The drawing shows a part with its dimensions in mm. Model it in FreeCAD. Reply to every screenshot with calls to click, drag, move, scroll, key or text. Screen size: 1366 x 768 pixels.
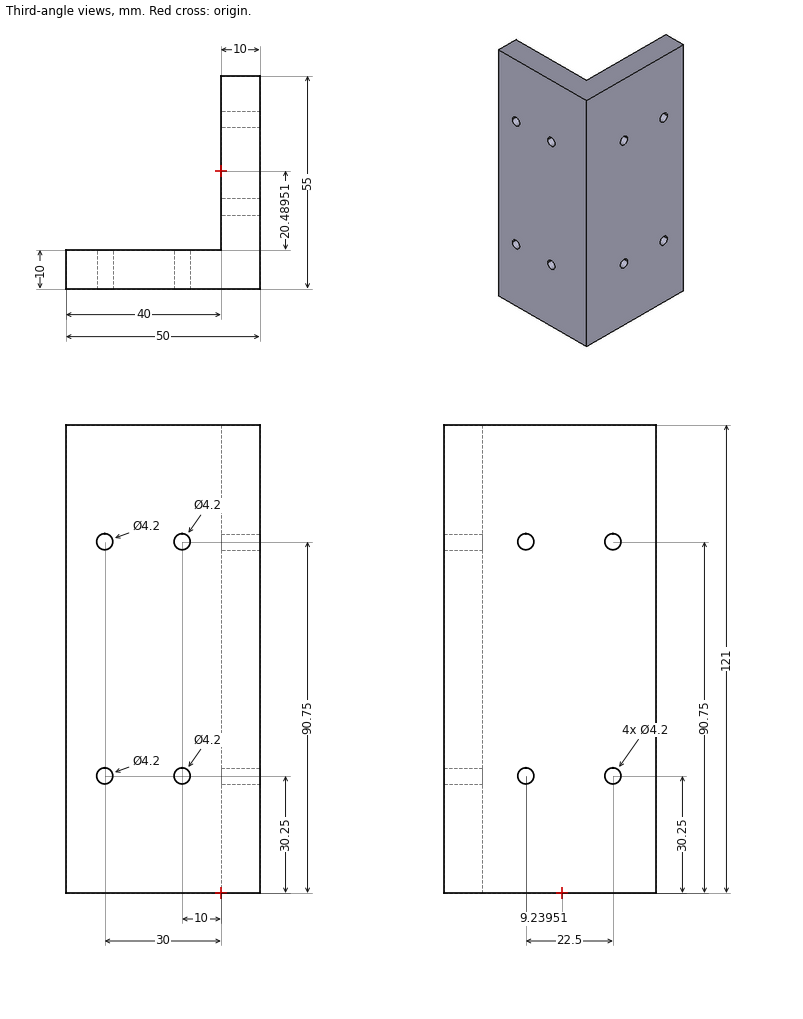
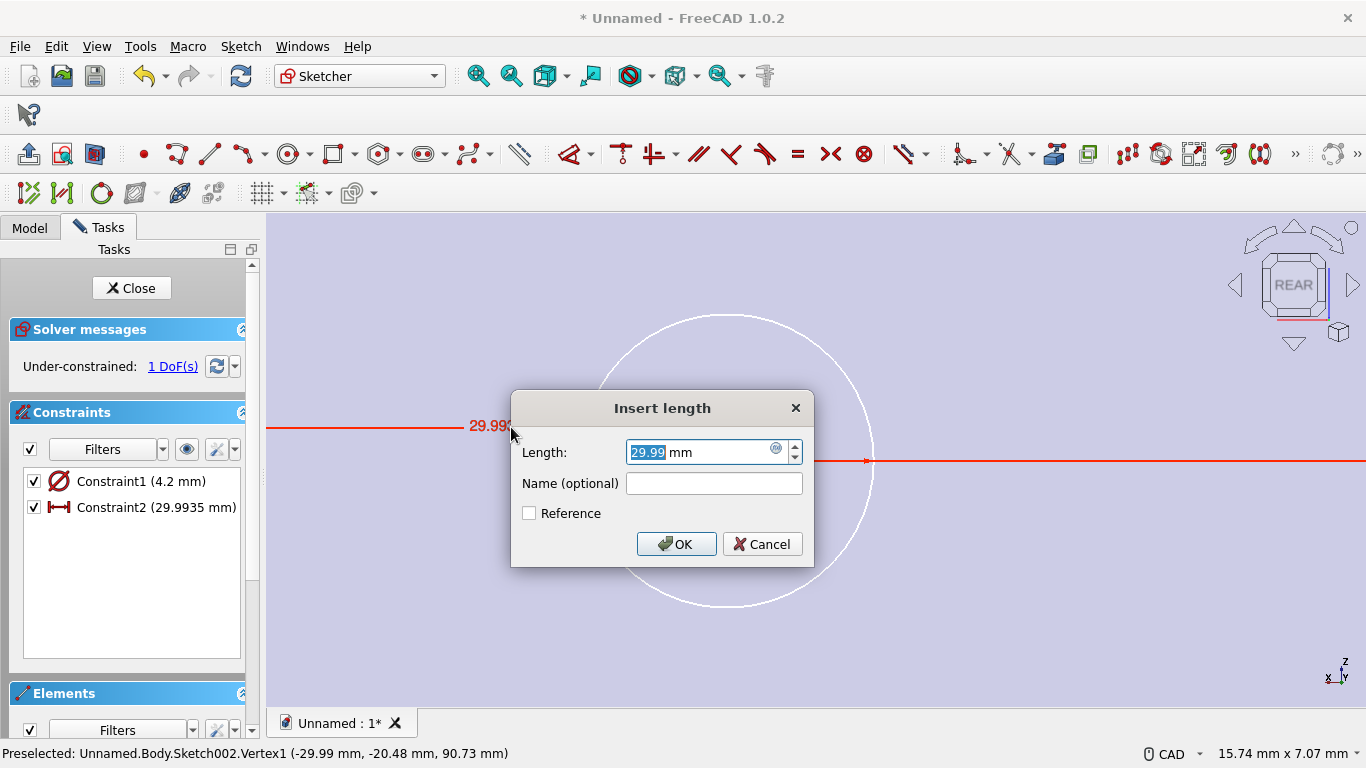
text(30)
key(Return)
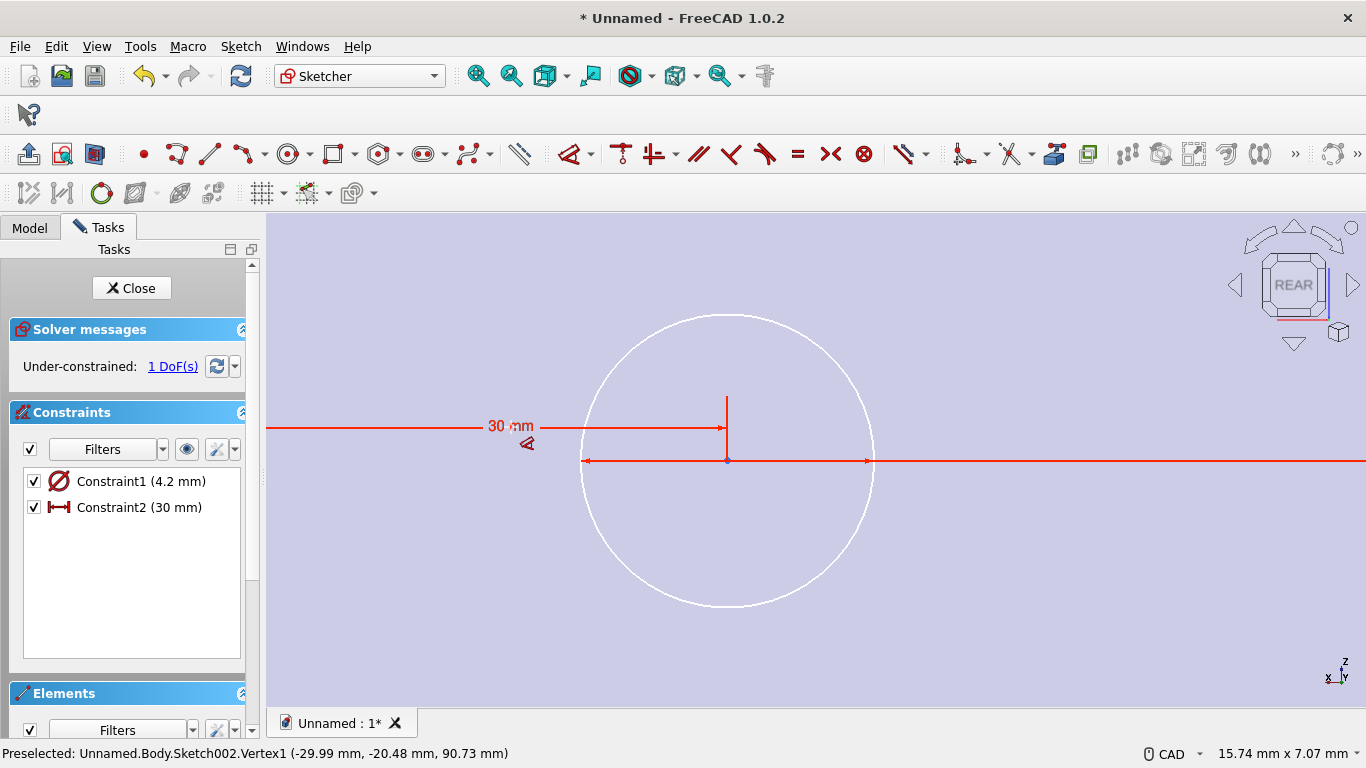
click(727, 461)
click(761, 570)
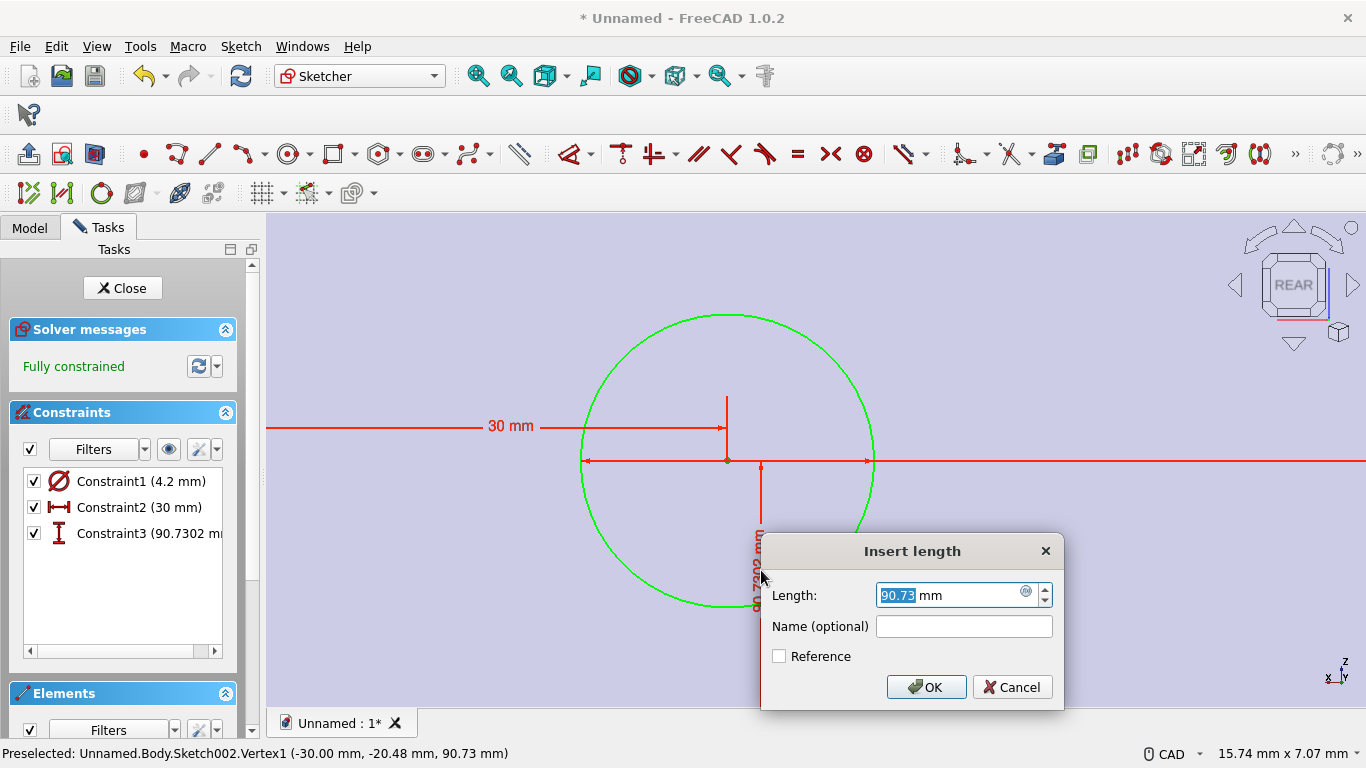
text(90.75)
key(Return)
key(Escape)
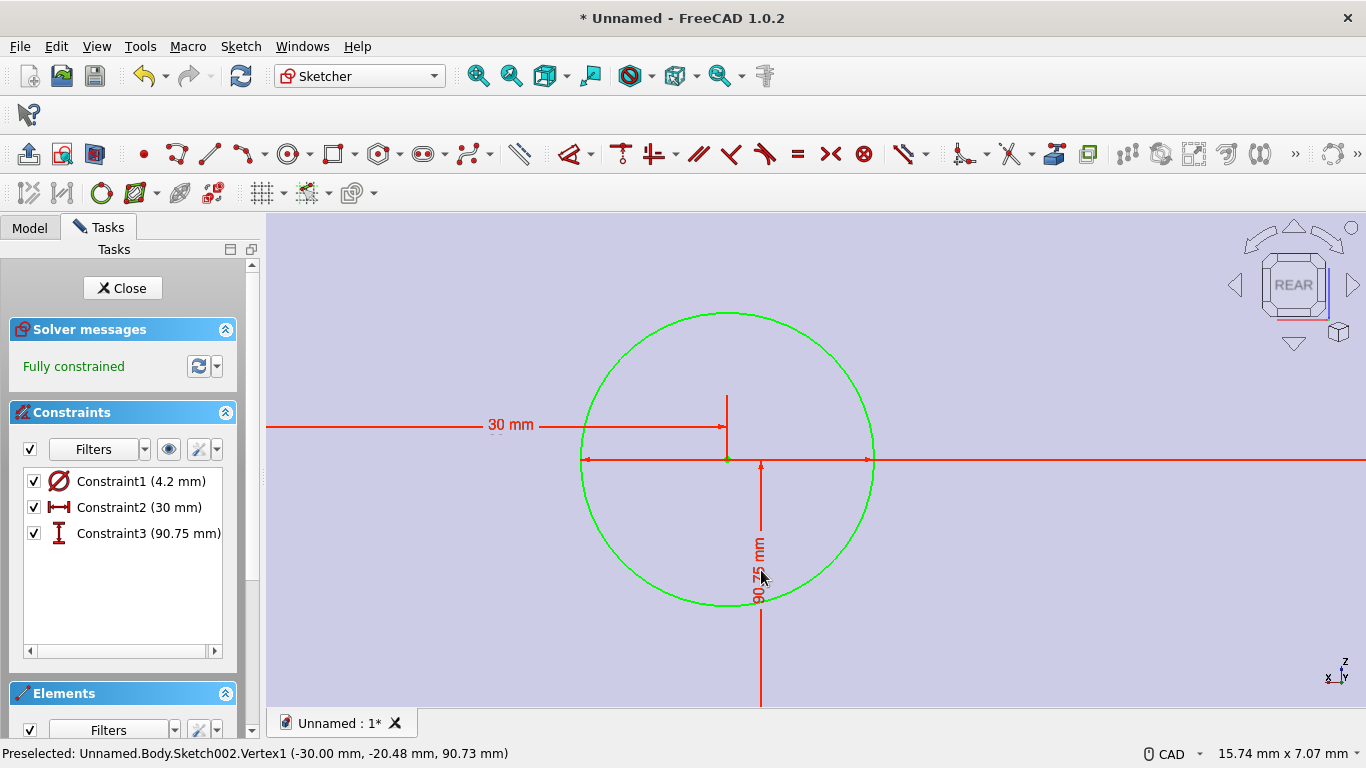
click(123, 288)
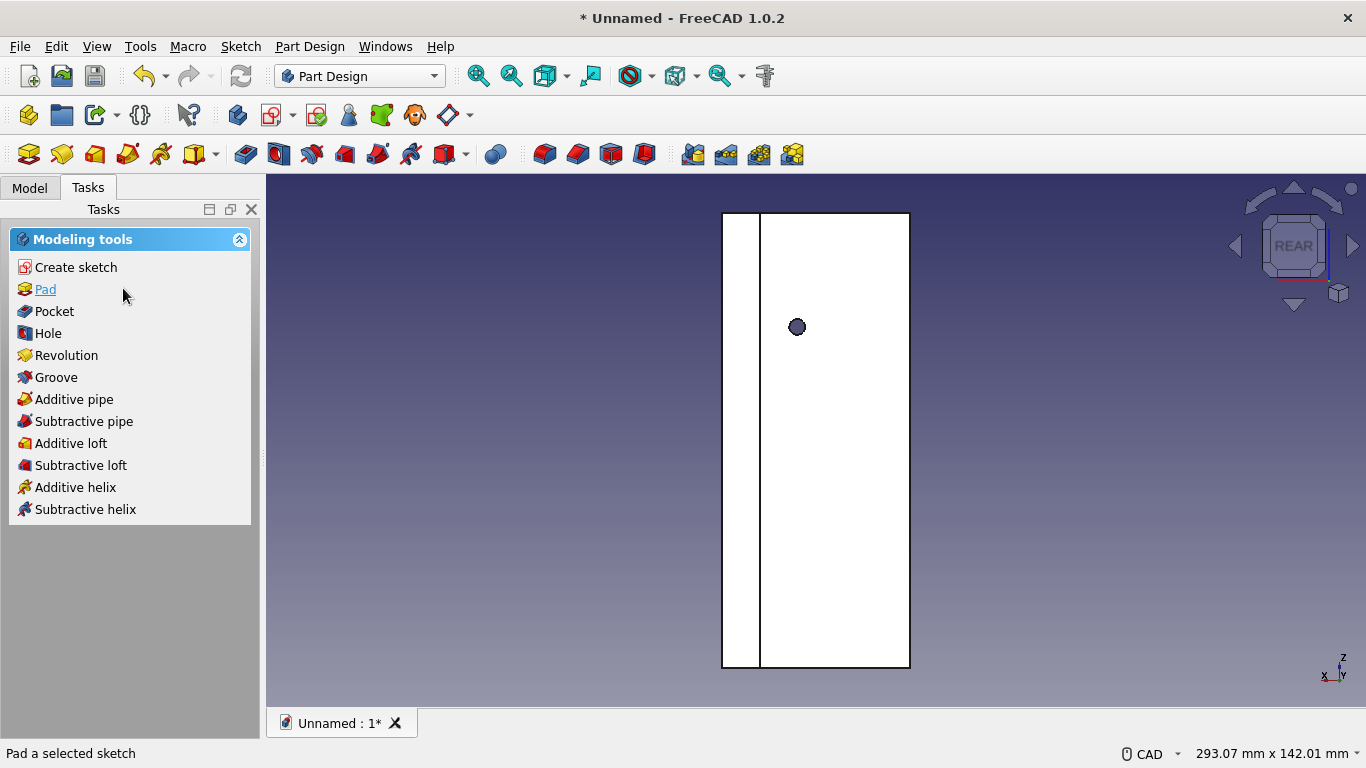
click(246, 154)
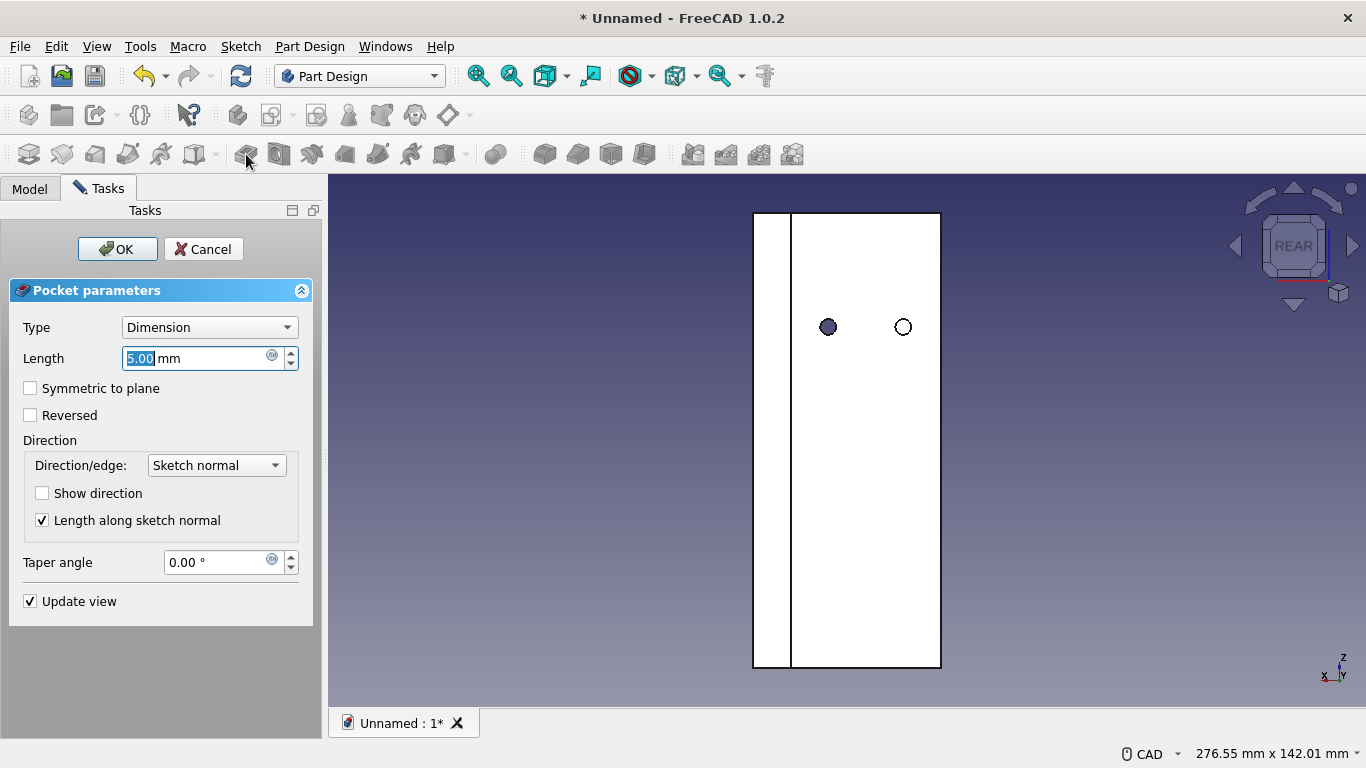
click(210, 328)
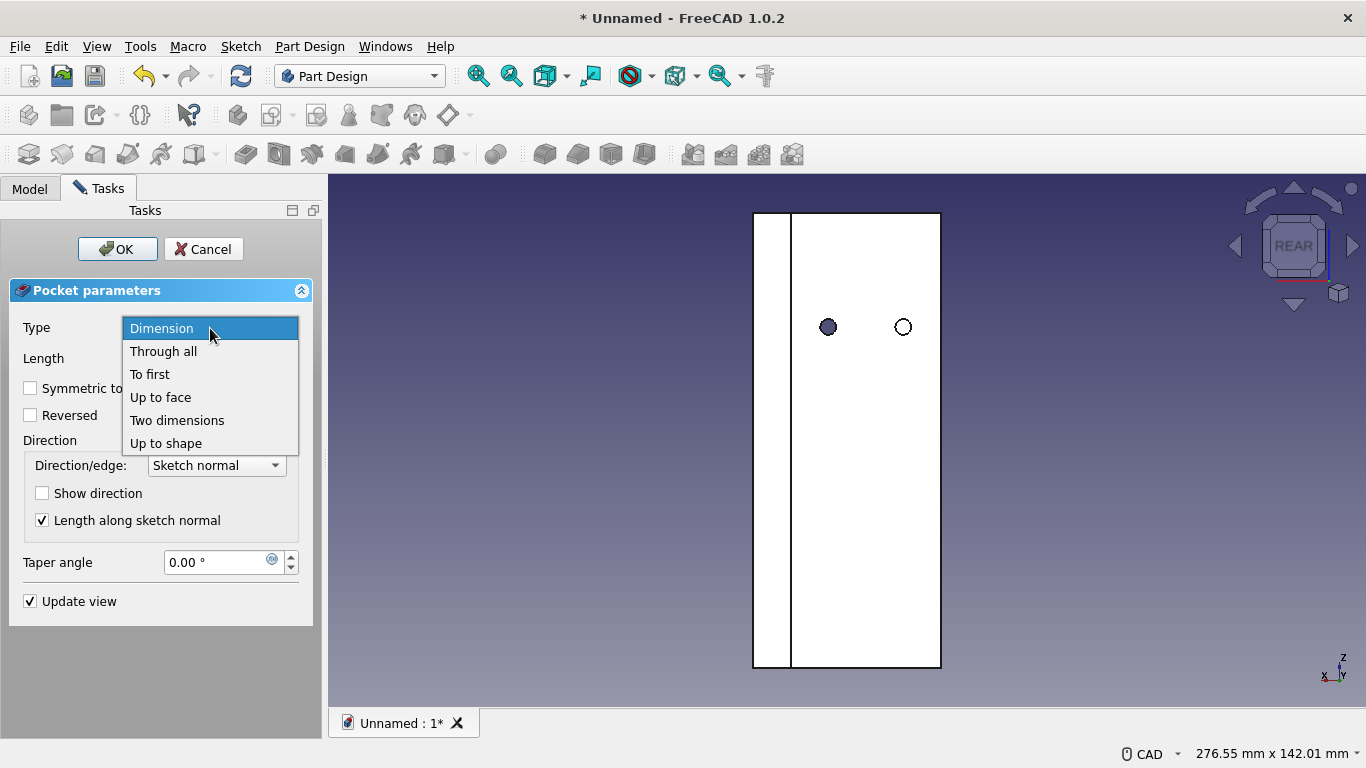
click(208, 374)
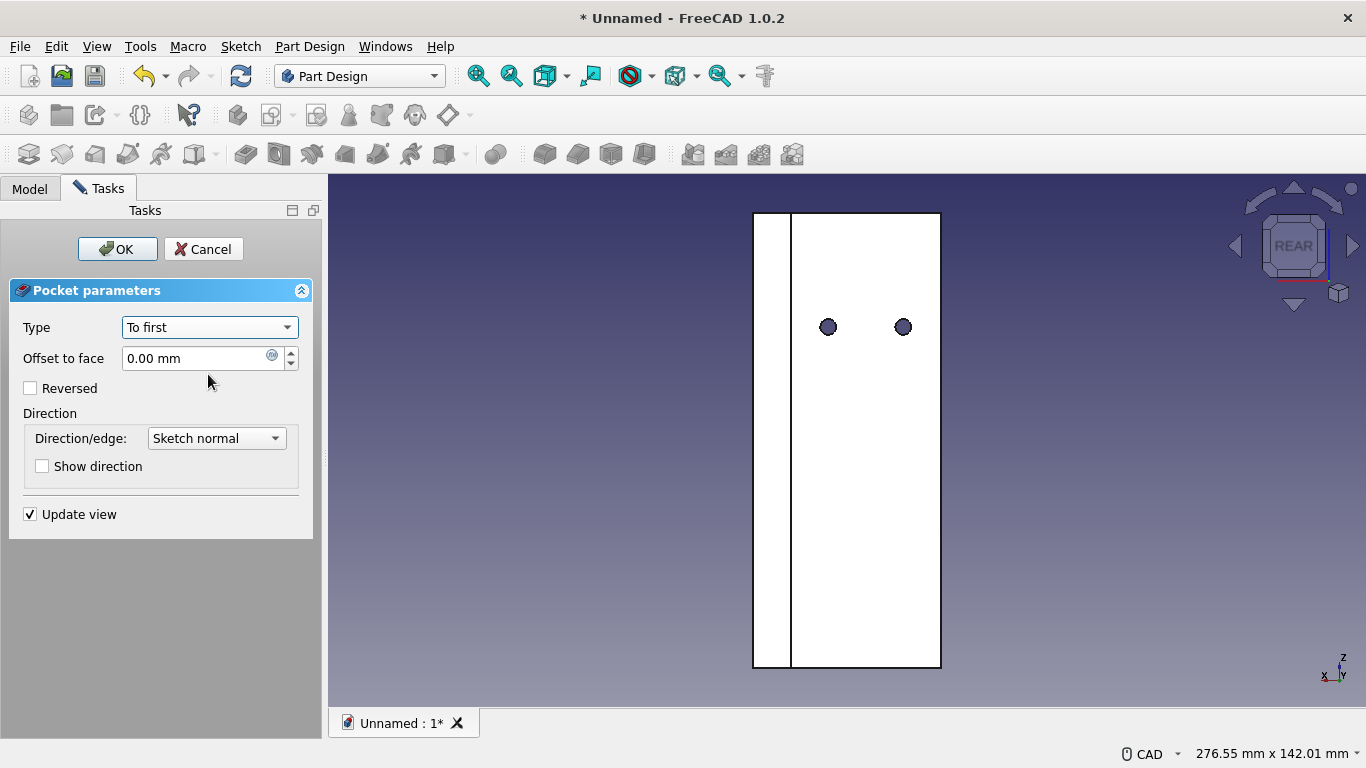
click(118, 249)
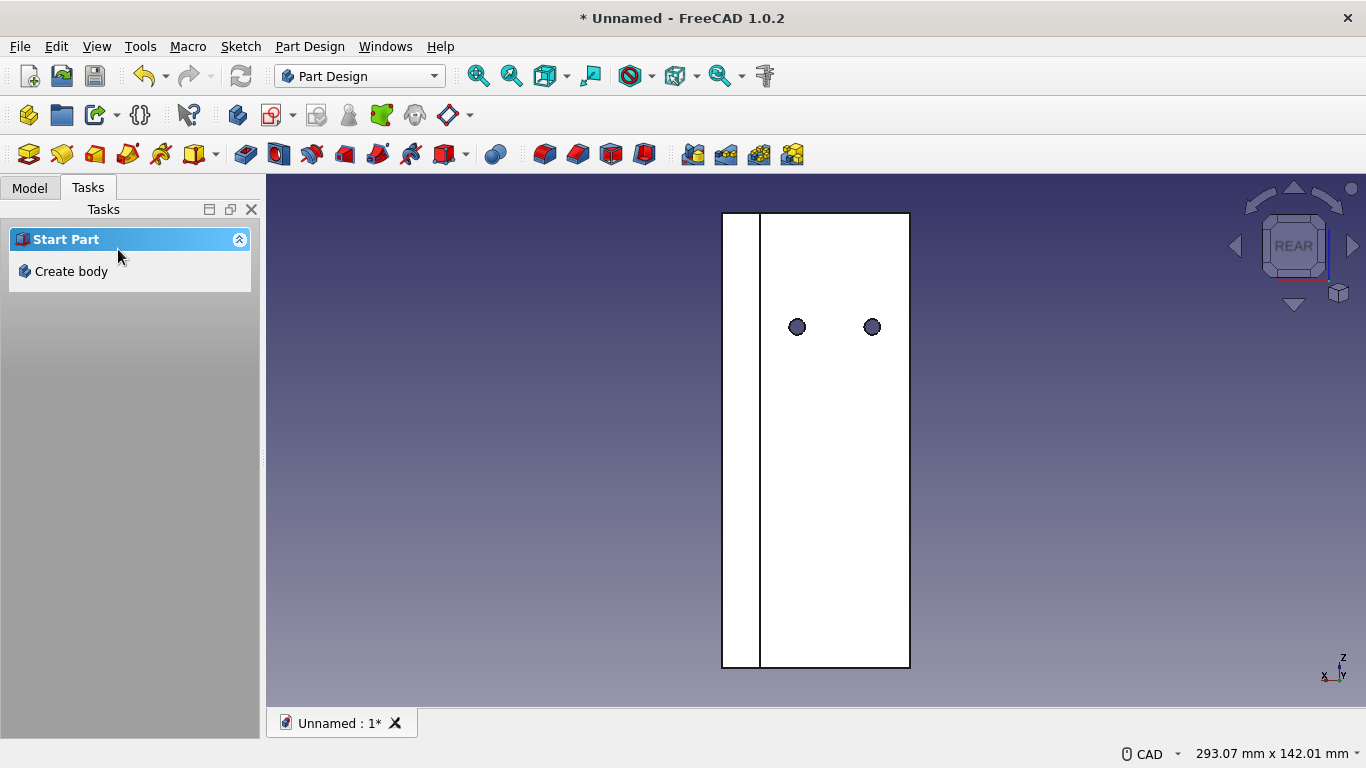
click(835, 439)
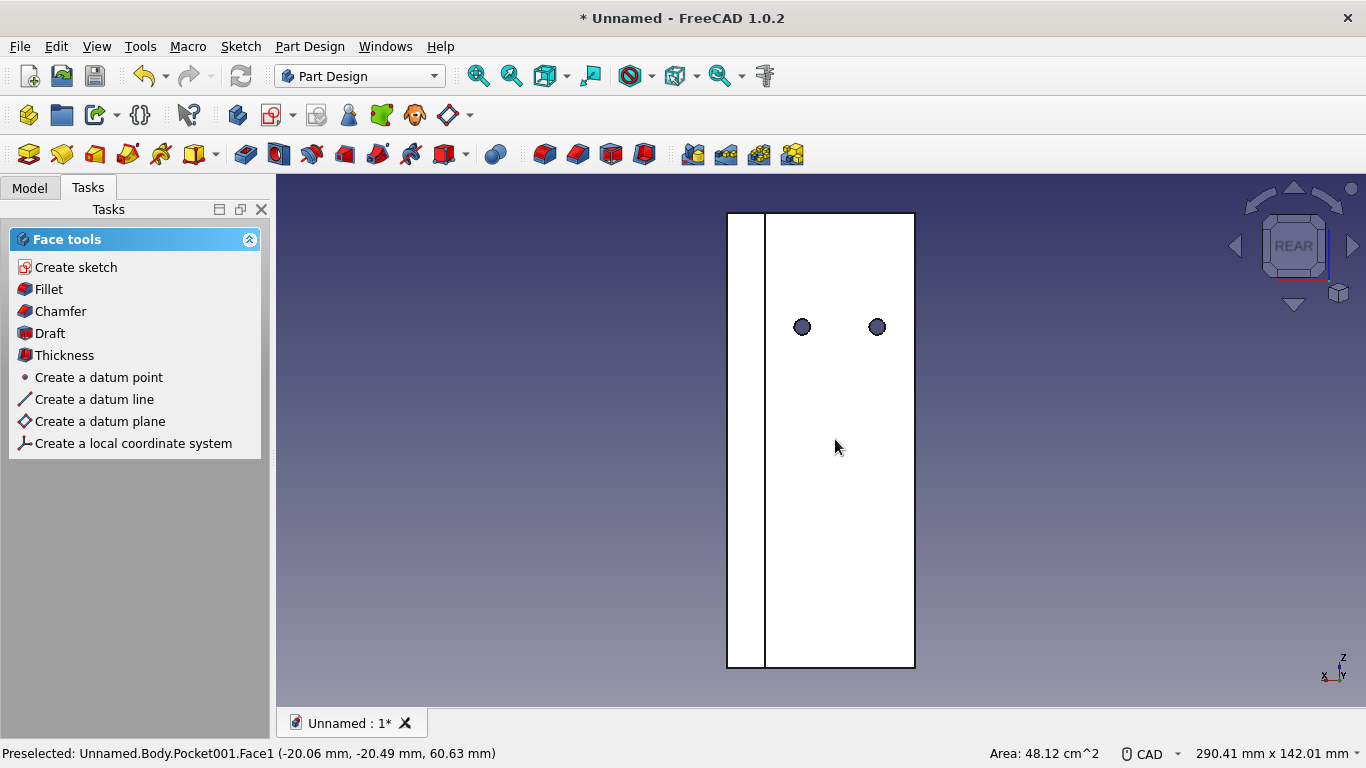
click(270, 116)